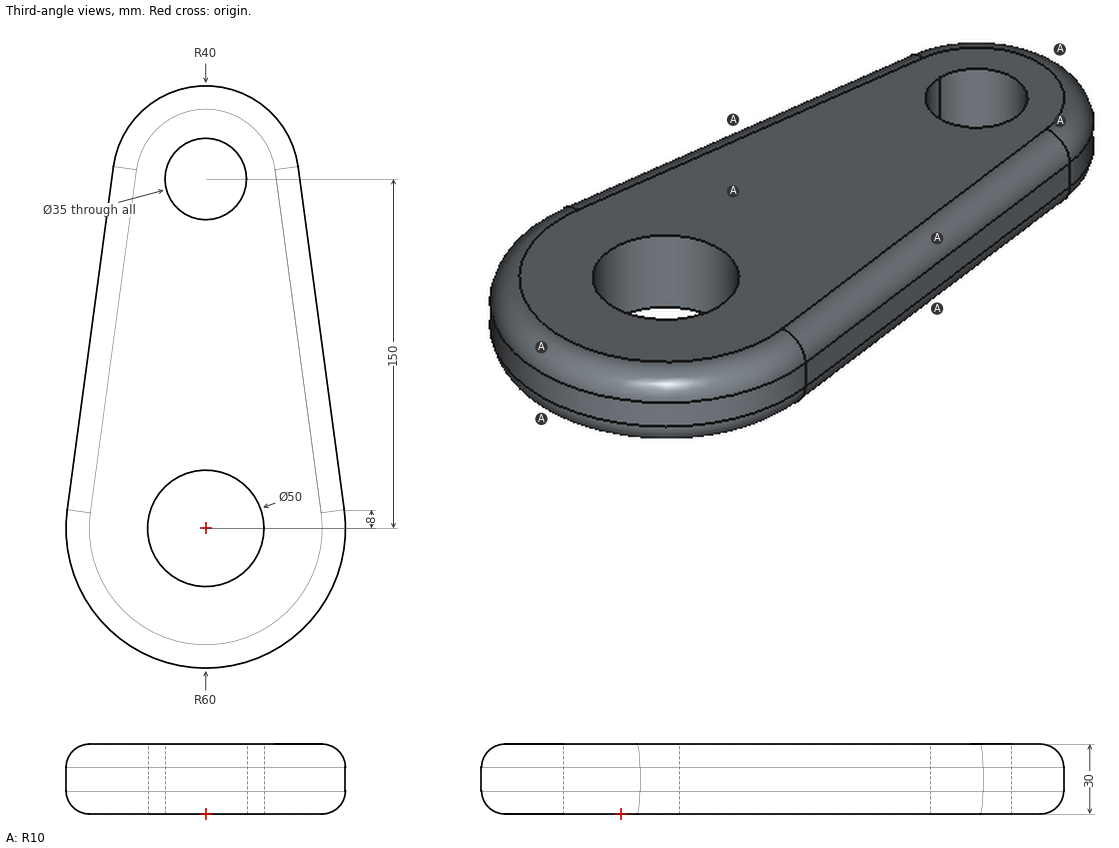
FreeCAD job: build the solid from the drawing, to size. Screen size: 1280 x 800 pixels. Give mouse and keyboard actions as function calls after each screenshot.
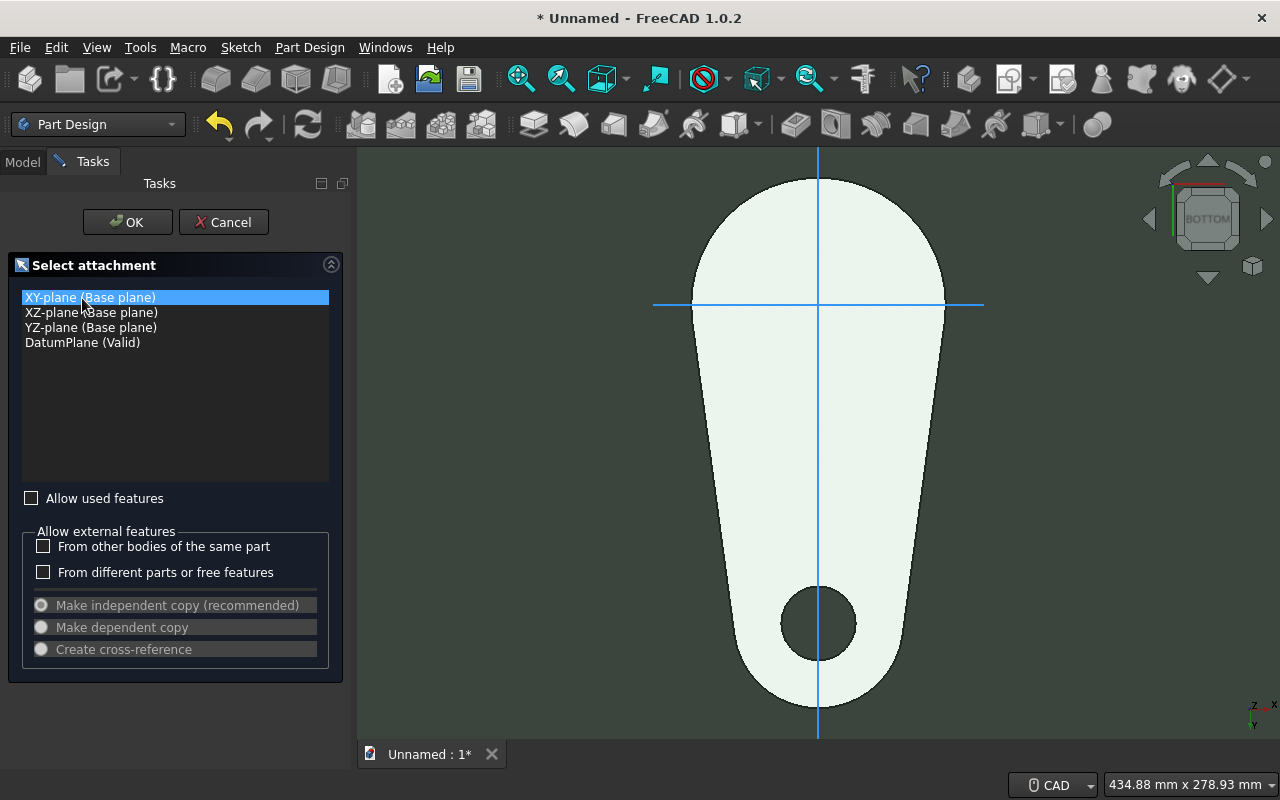
click(128, 222)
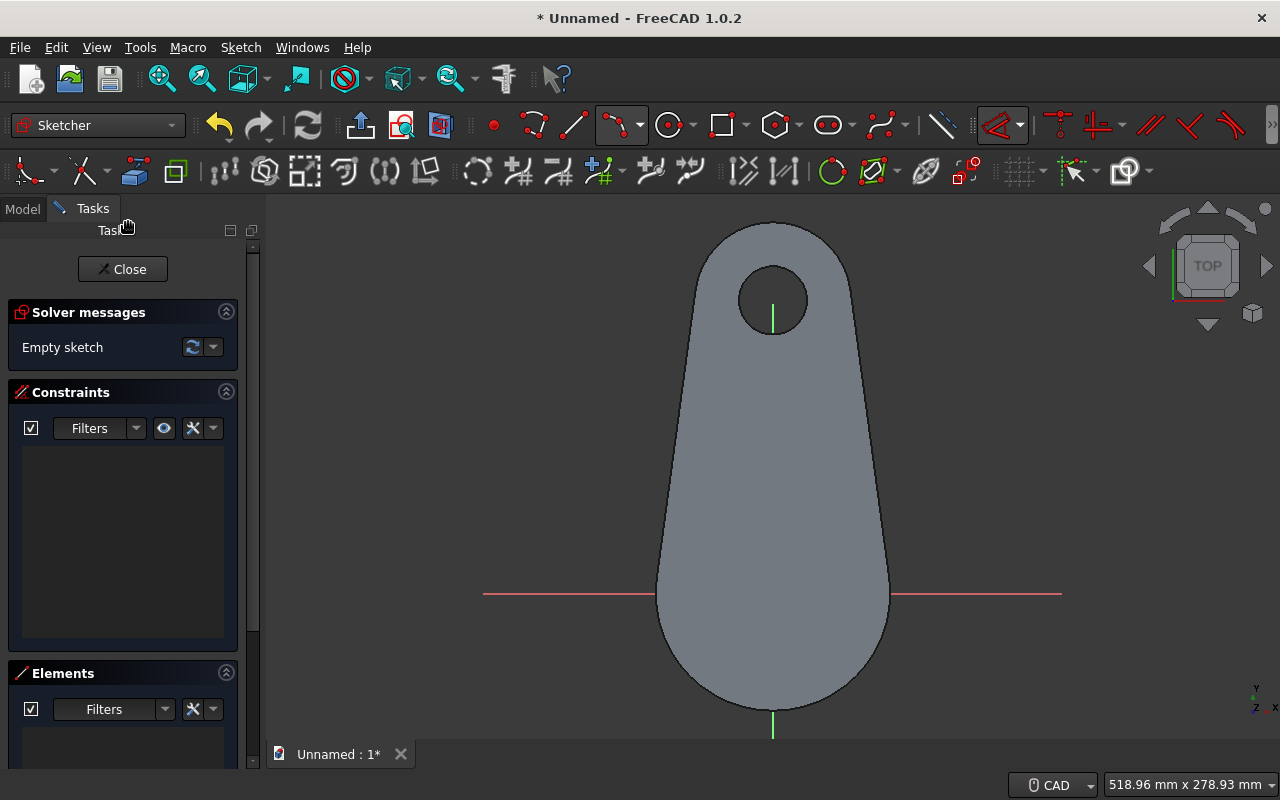
click(442, 126)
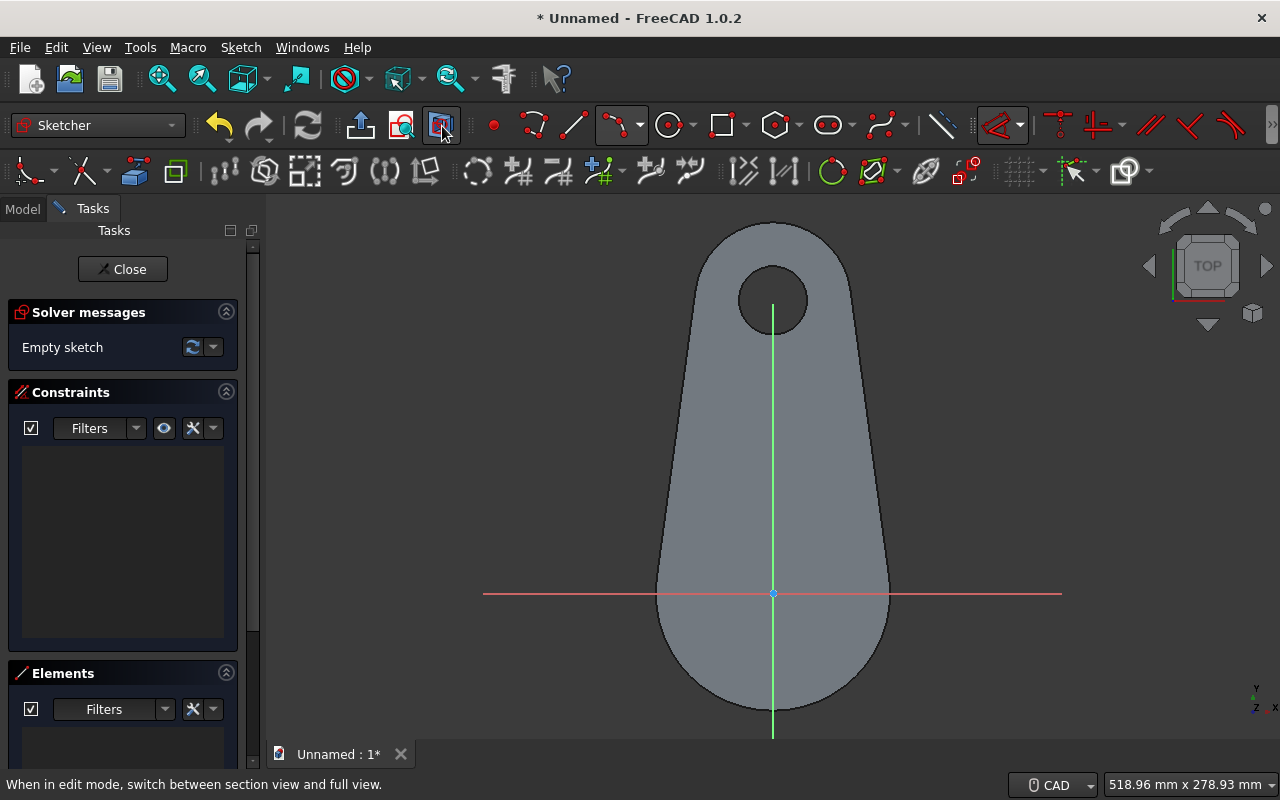
scroll(803, 648, up, 6)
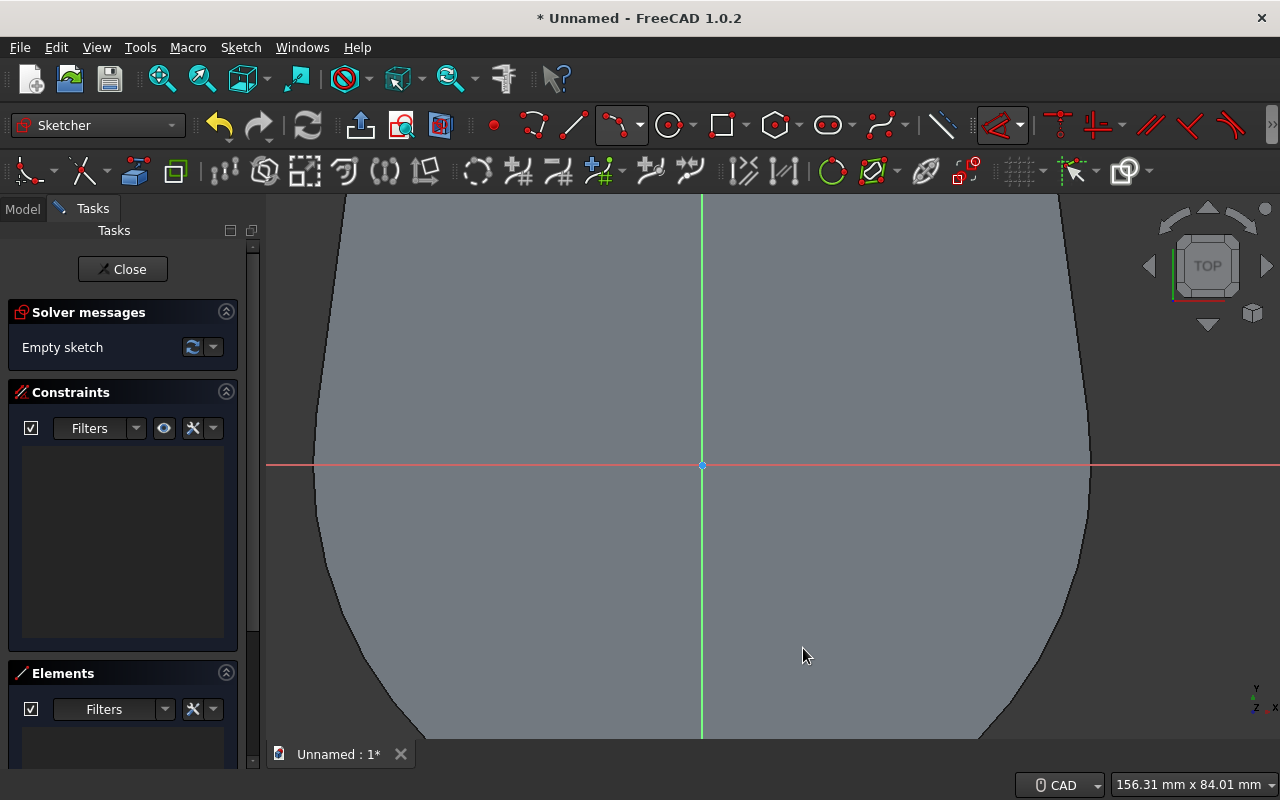
click(670, 126)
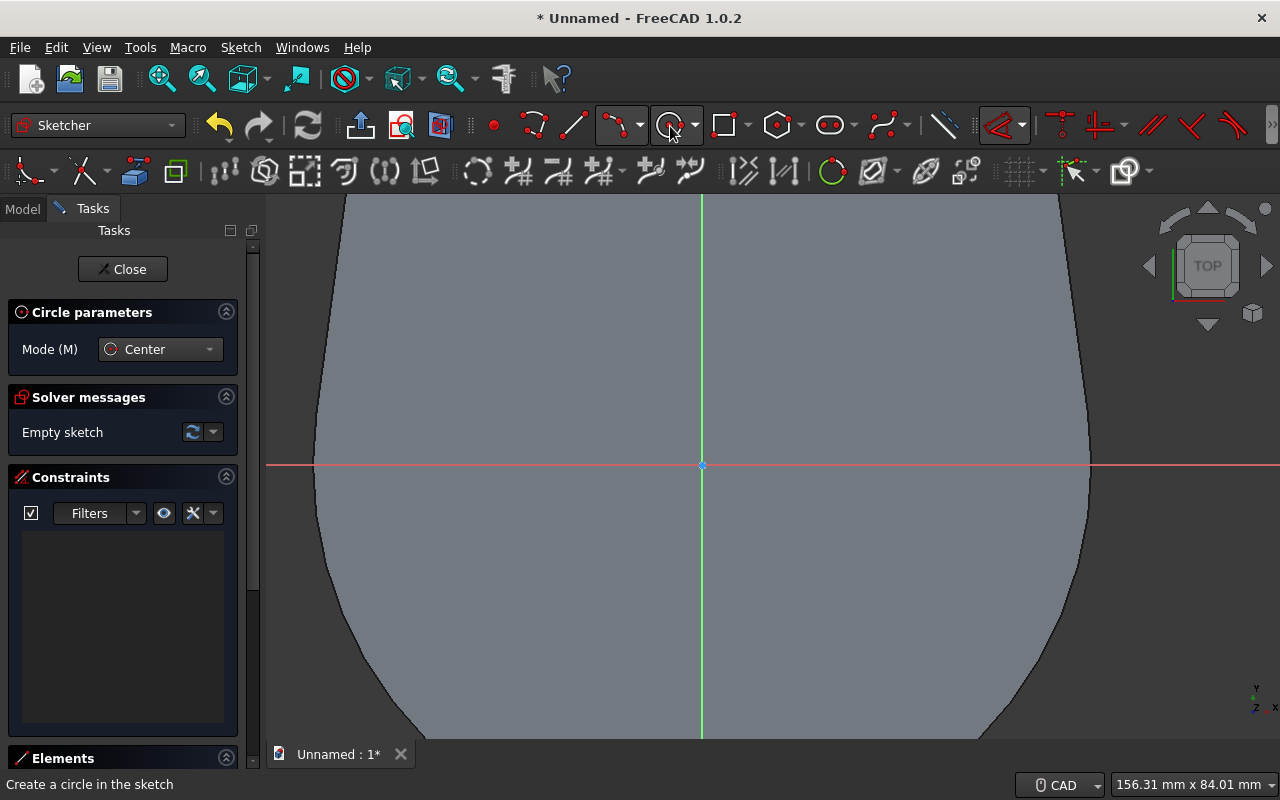
click(702, 465)
click(817, 350)
key(Escape)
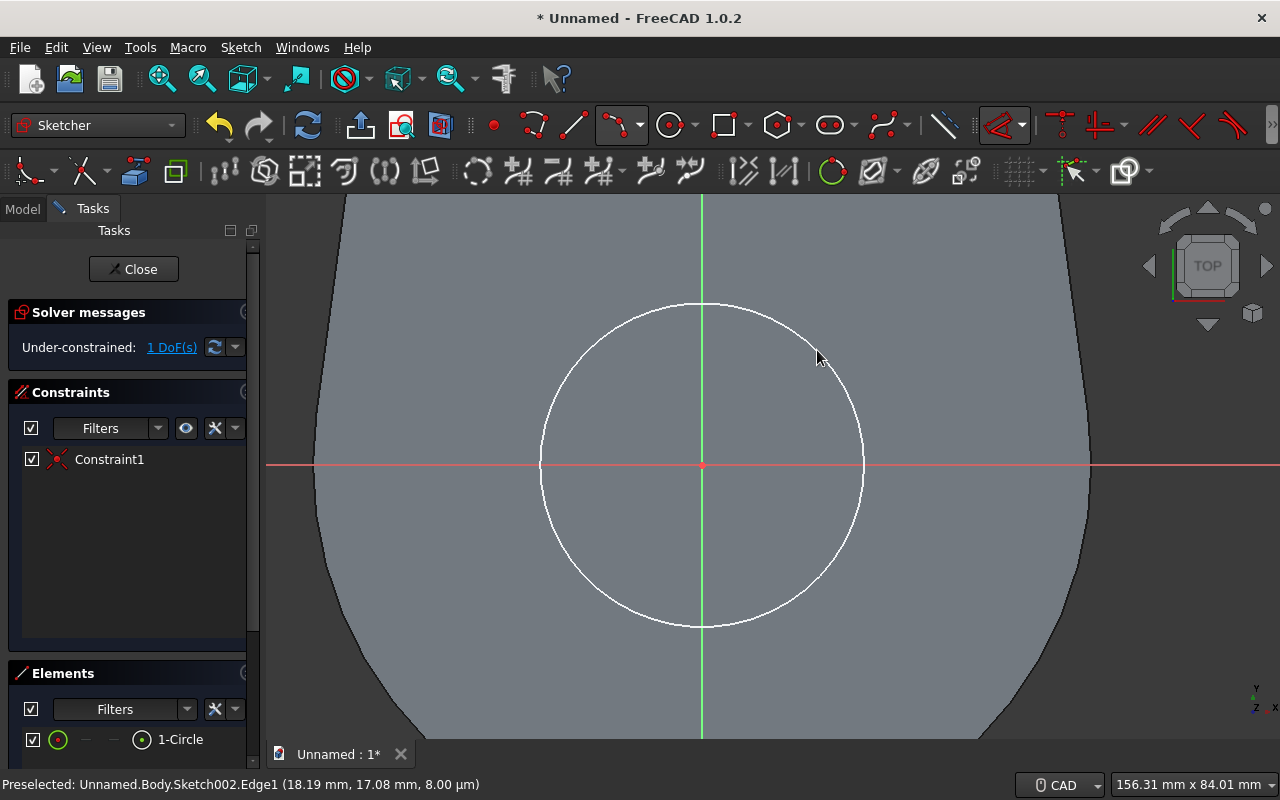
click(816, 350)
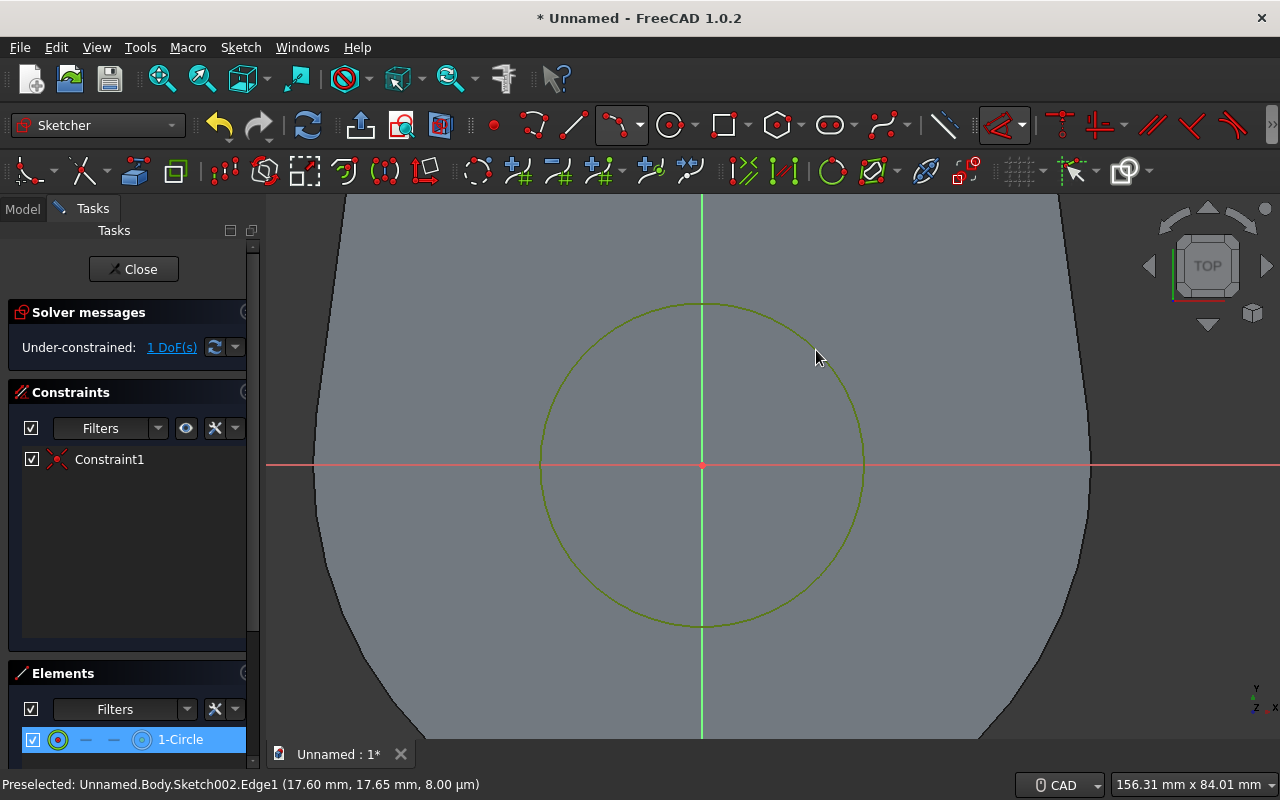
click(1024, 126)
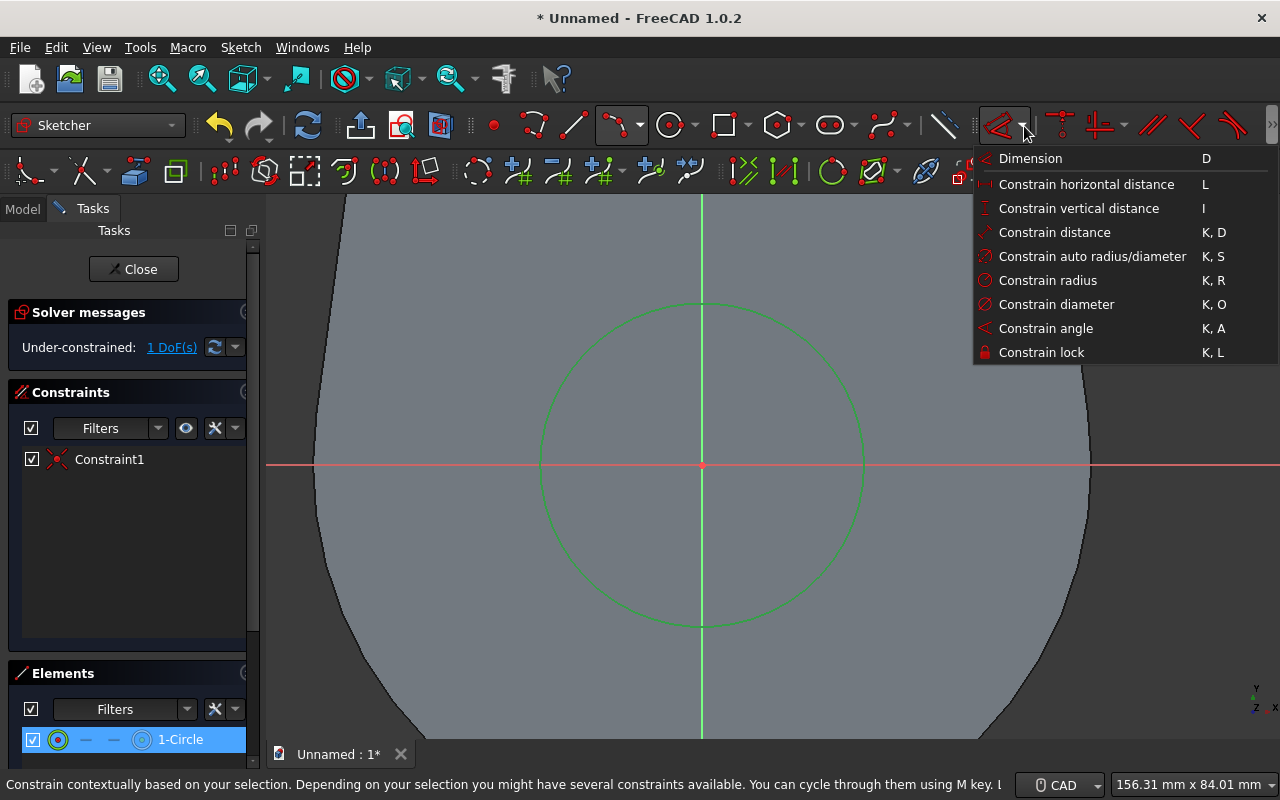
click(1126, 304)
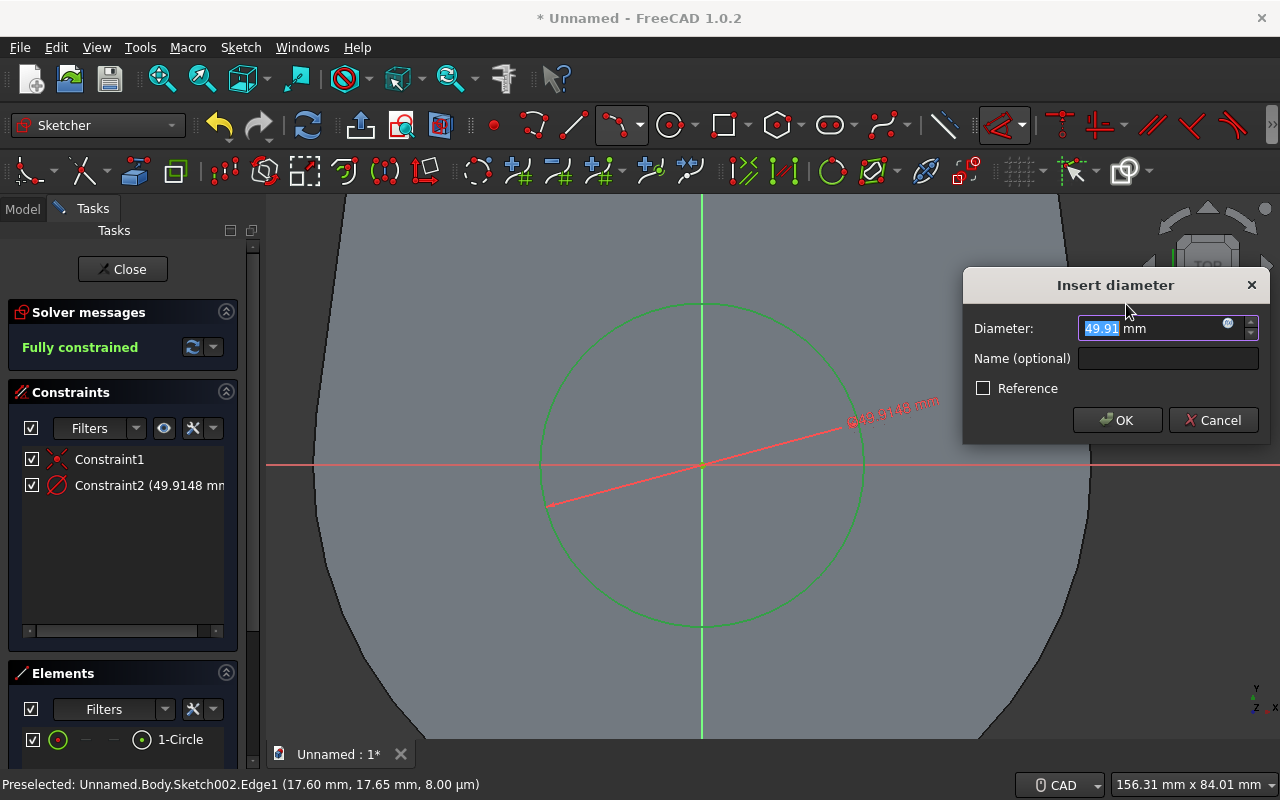
text(50)
key(Return)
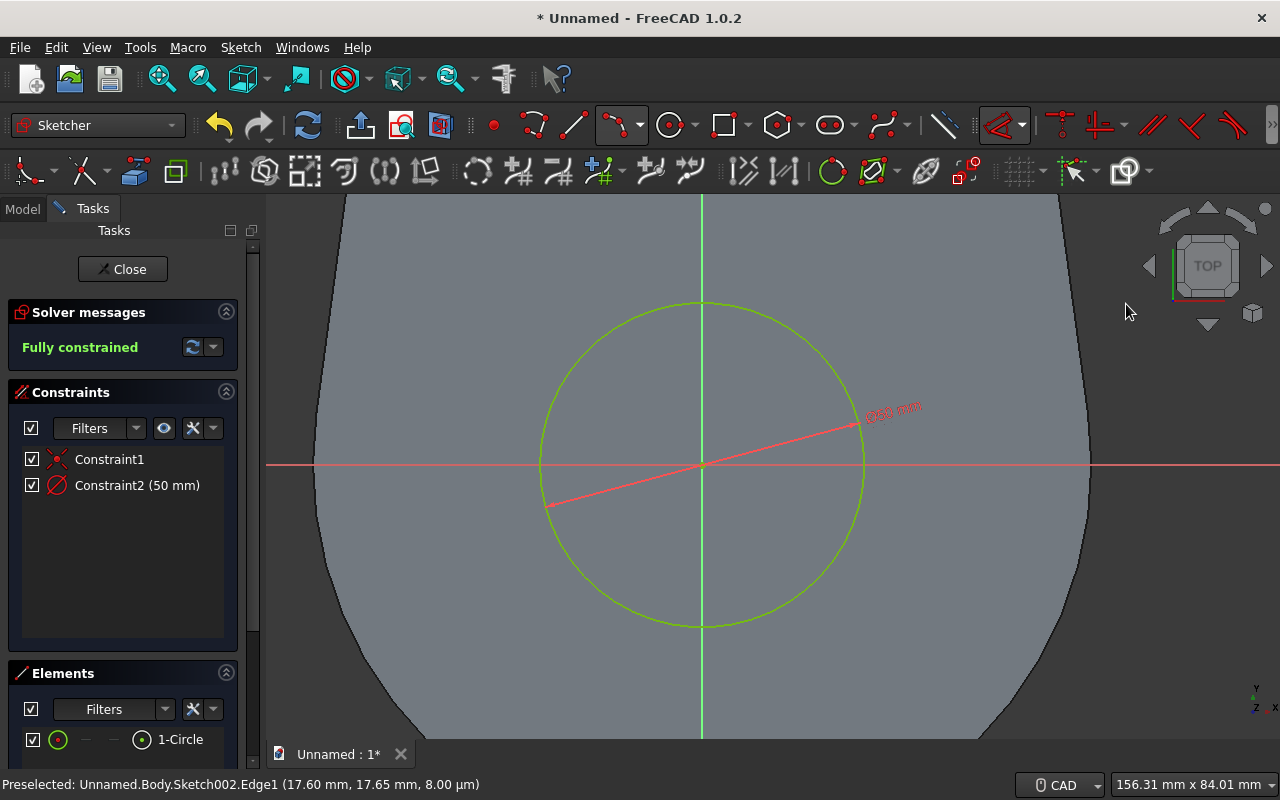
click(123, 269)